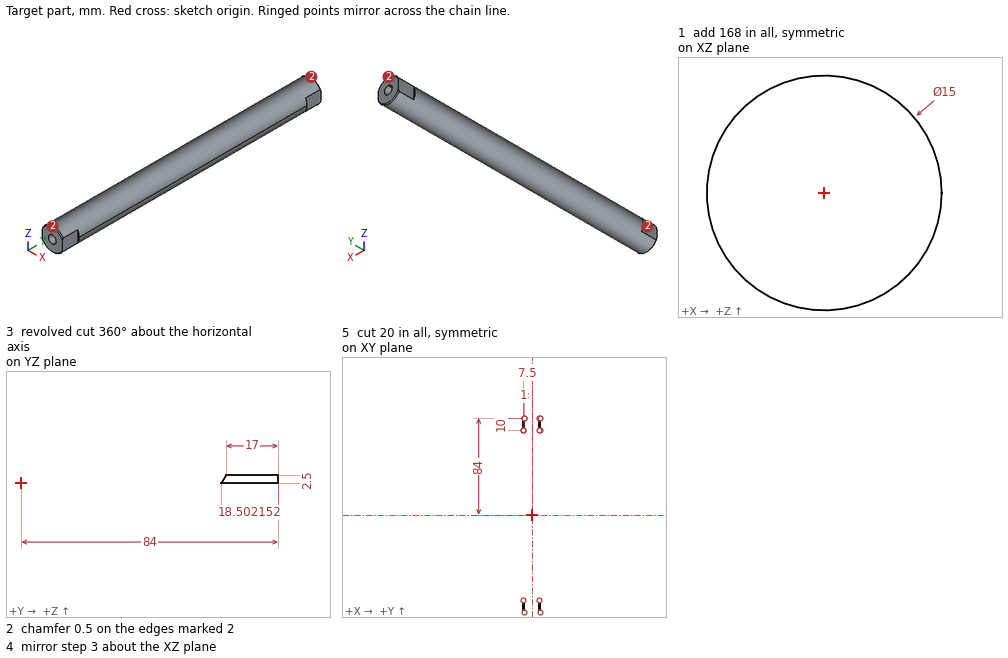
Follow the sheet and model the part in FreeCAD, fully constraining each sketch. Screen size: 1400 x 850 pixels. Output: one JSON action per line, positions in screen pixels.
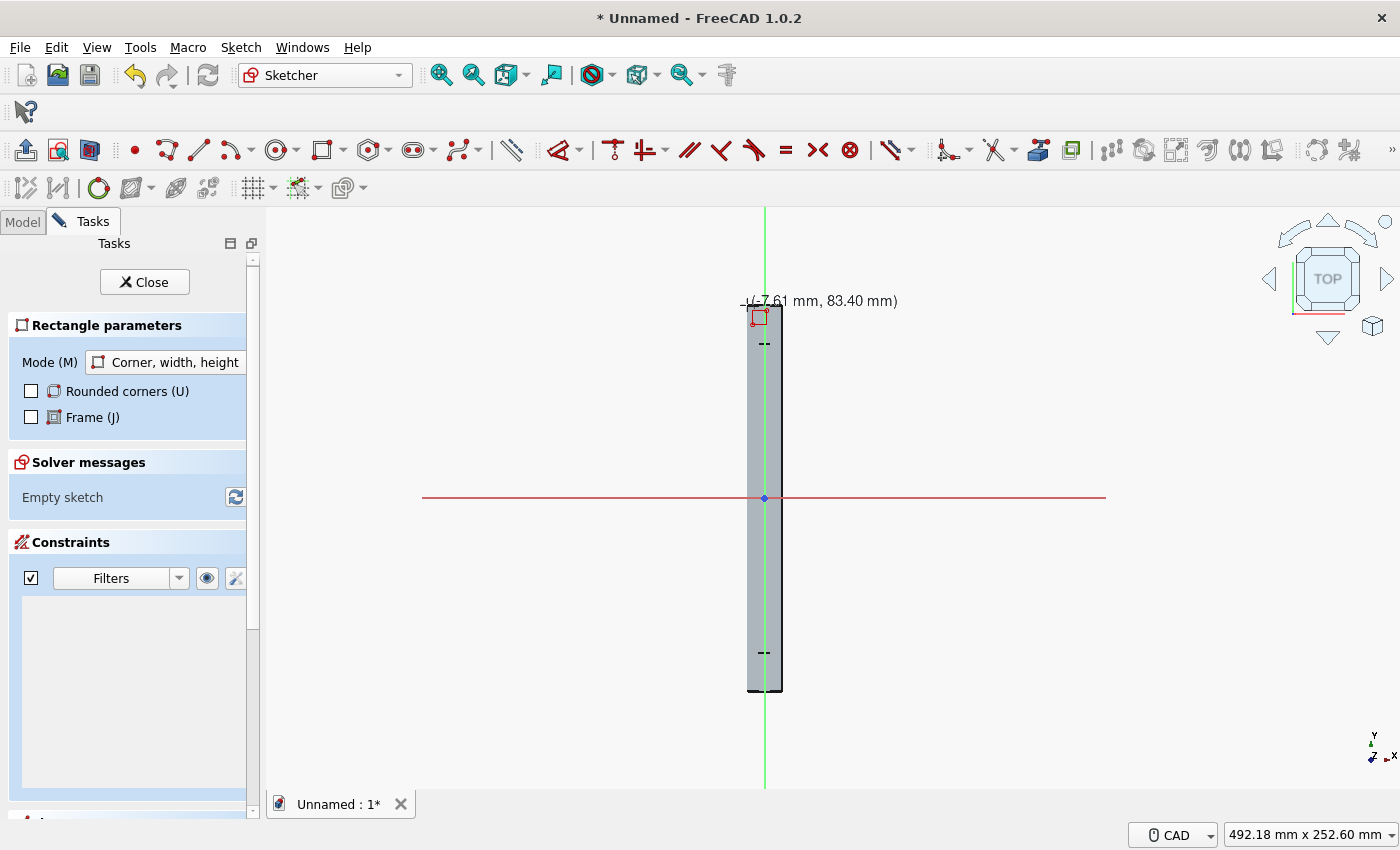
{"action": "left_click", "coordinate": [747, 305]}
{"action": "left_click", "coordinate": [750, 328]}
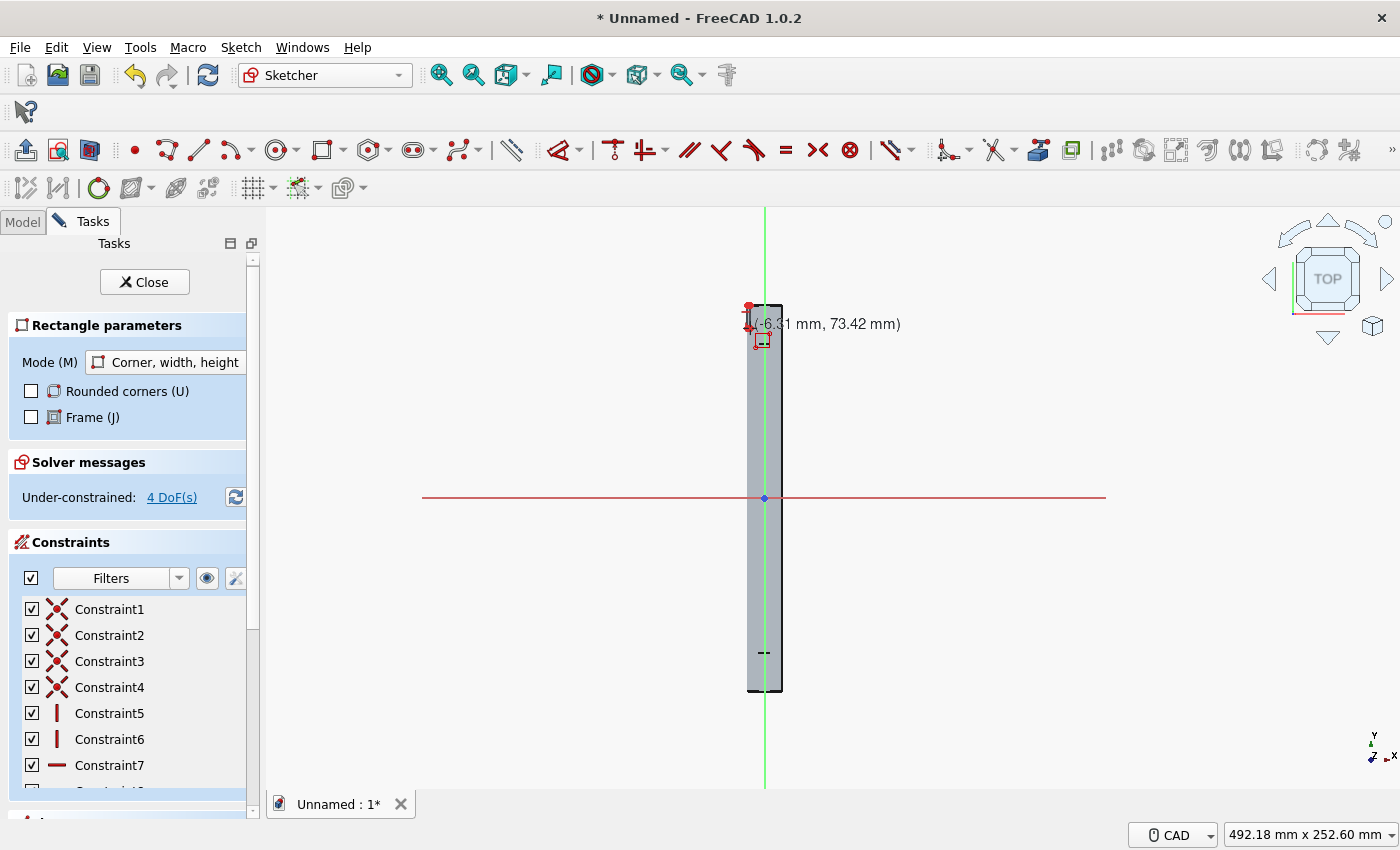
{"action": "scroll", "coordinate": [780, 305], "scroll_direction": "up", "scroll_amount": 10}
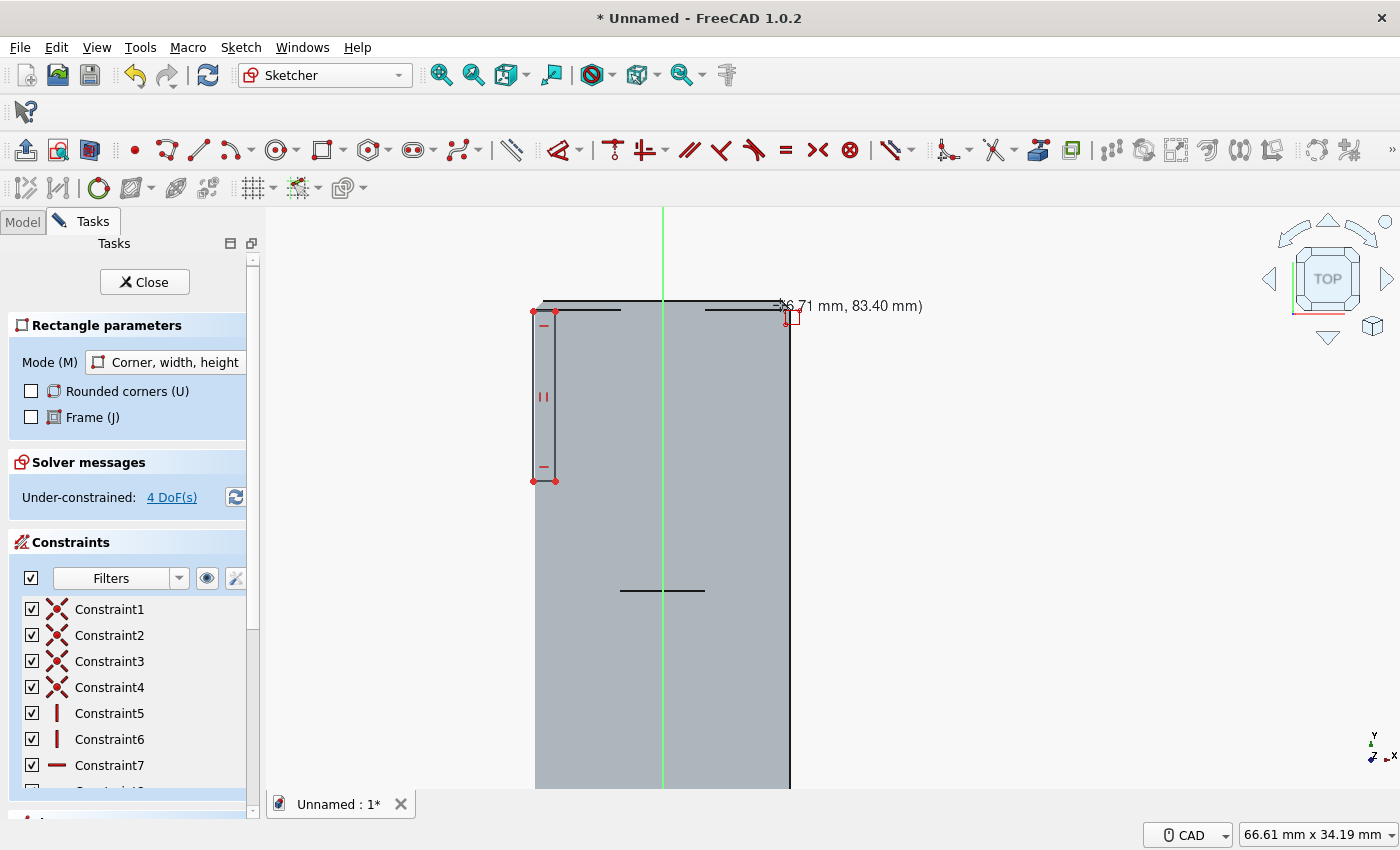
{"action": "scroll", "coordinate": [780, 305], "scroll_direction": "down", "scroll_amount": 10}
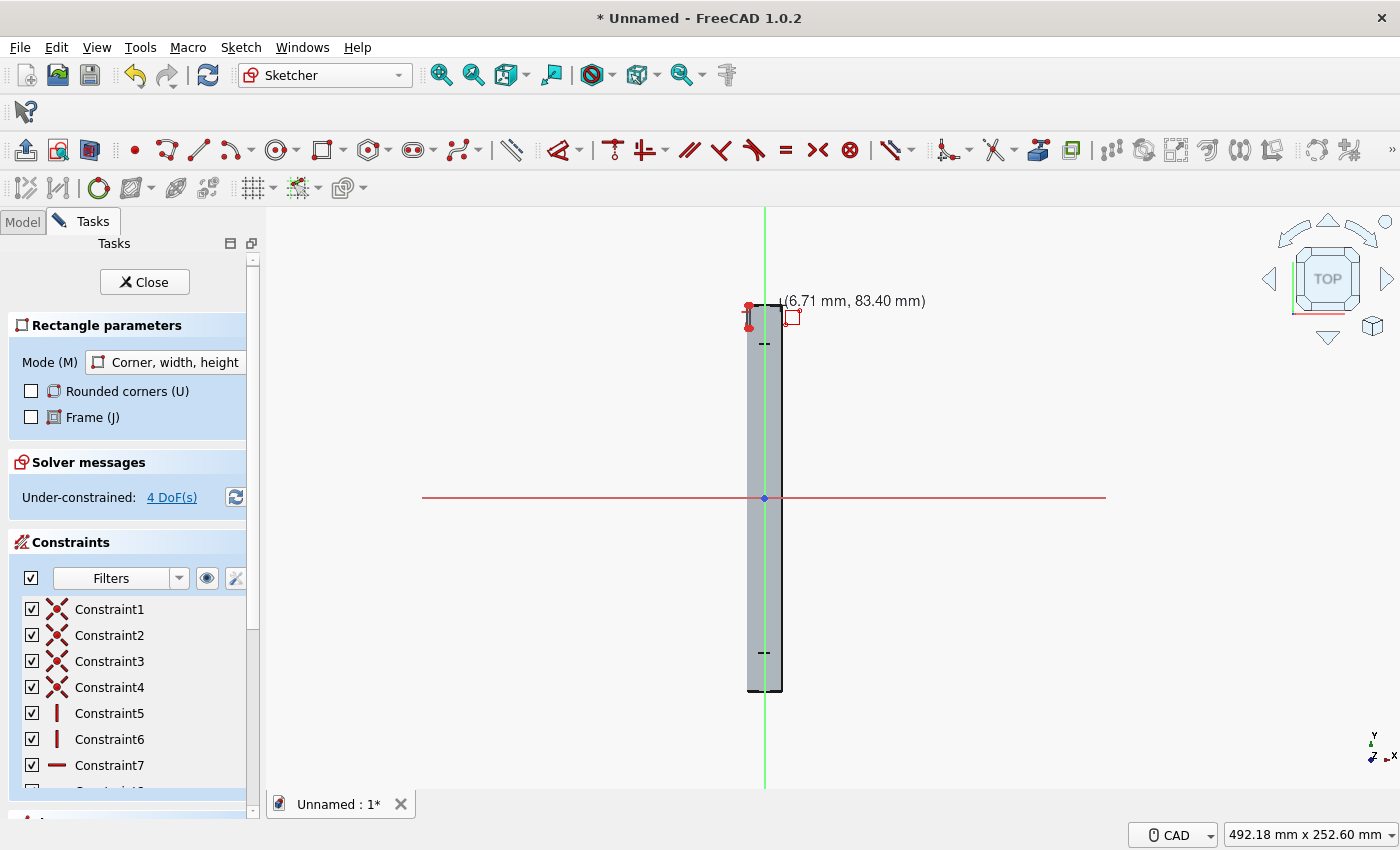
{"action": "left_click", "coordinate": [780, 305]}
{"action": "left_click", "coordinate": [782, 328]}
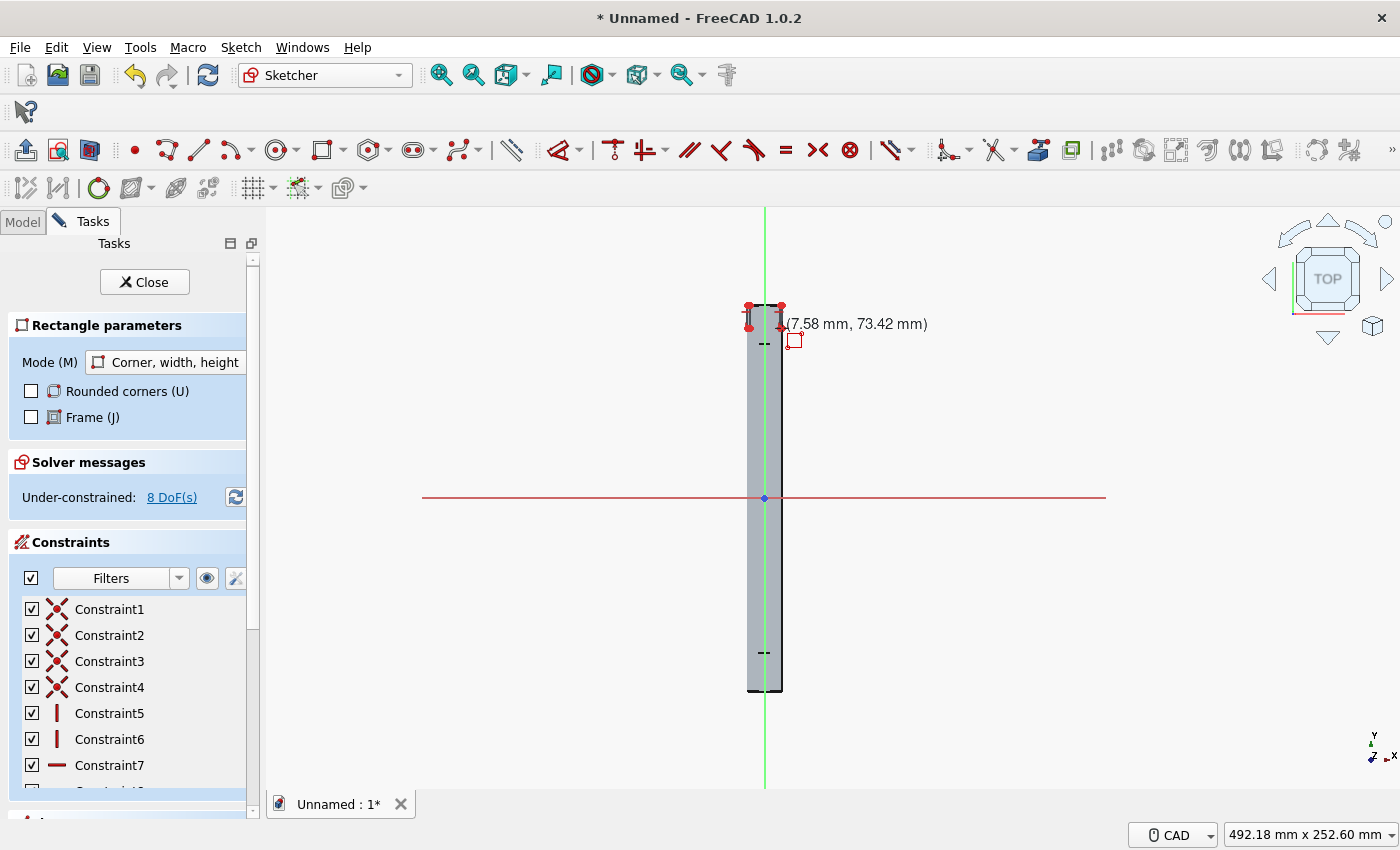
{"action": "scroll", "coordinate": [780, 669], "scroll_direction": "up", "scroll_amount": 10}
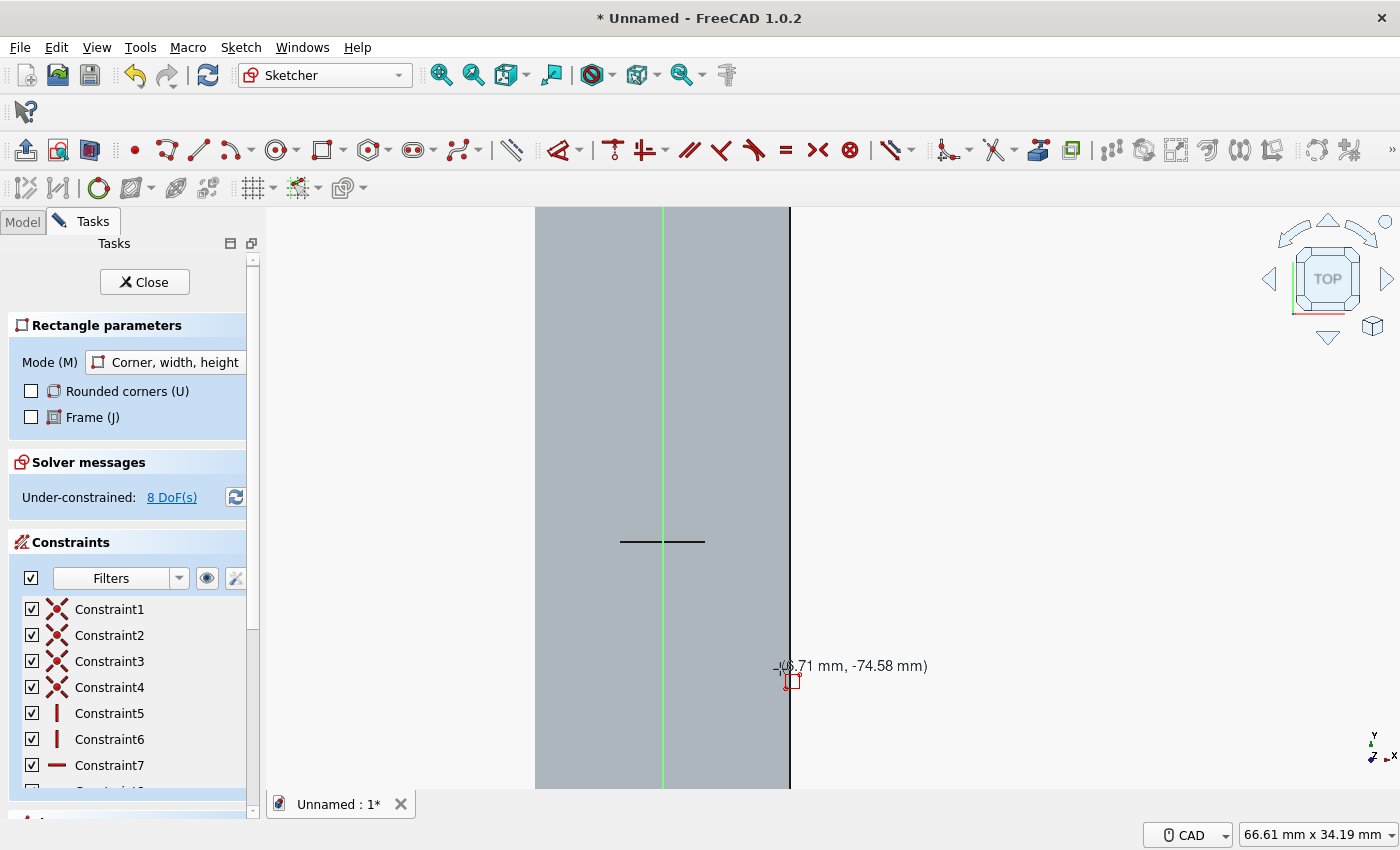
{"action": "scroll", "coordinate": [780, 670], "scroll_direction": "down", "scroll_amount": 10}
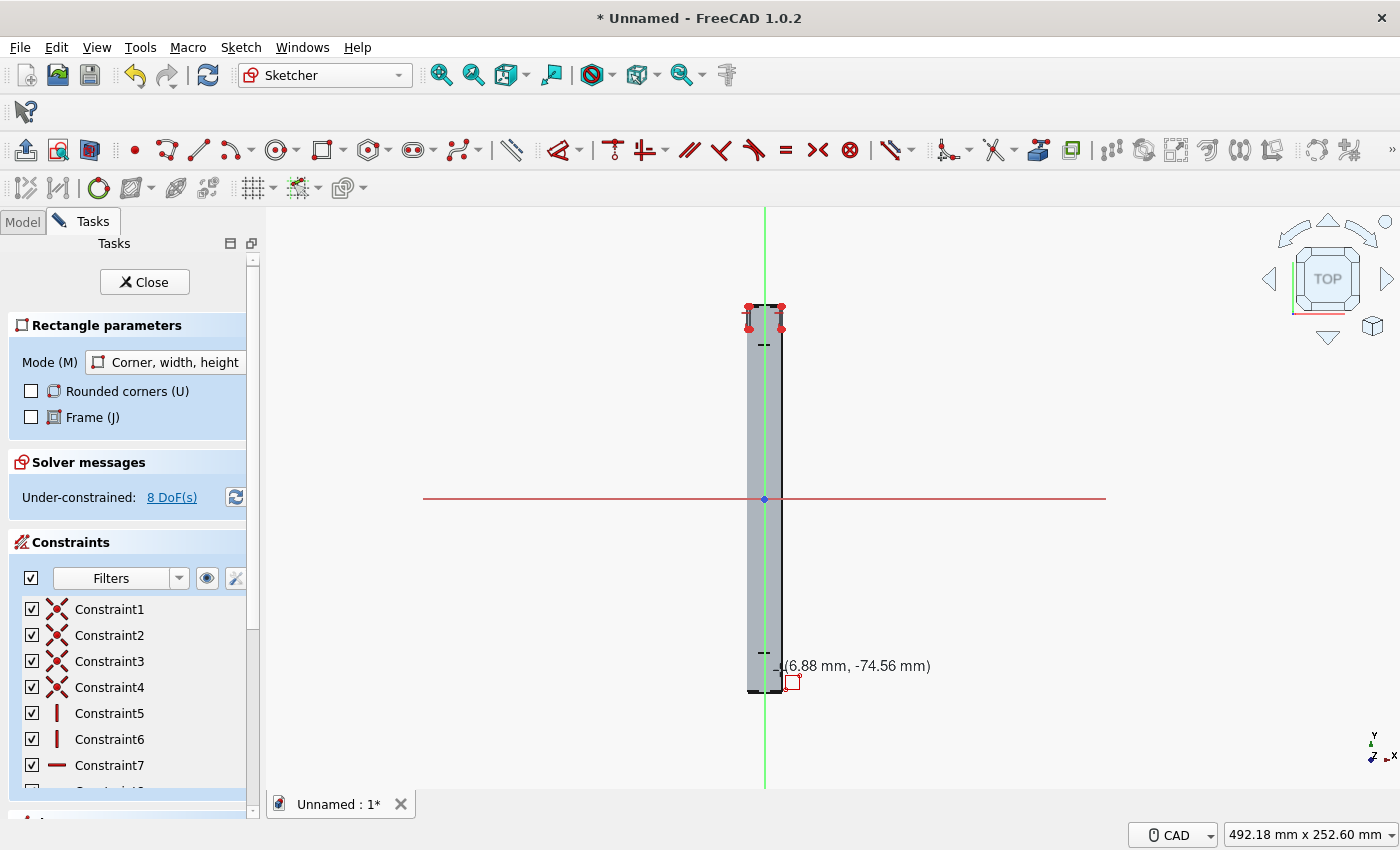
{"action": "left_click", "coordinate": [780, 670]}
{"action": "left_click", "coordinate": [782, 693]}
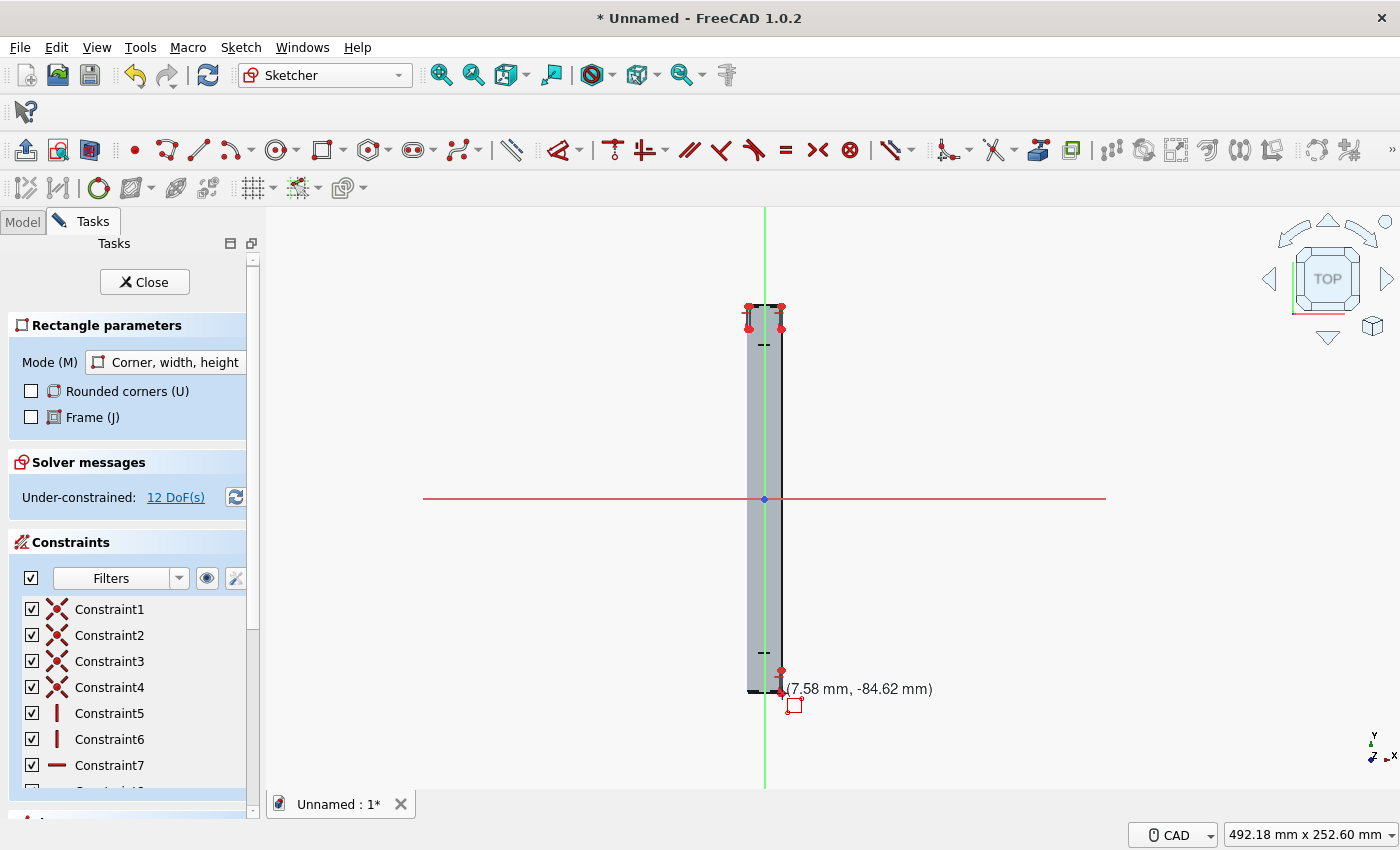
{"action": "scroll", "coordinate": [747, 670], "scroll_direction": "up", "scroll_amount": 10}